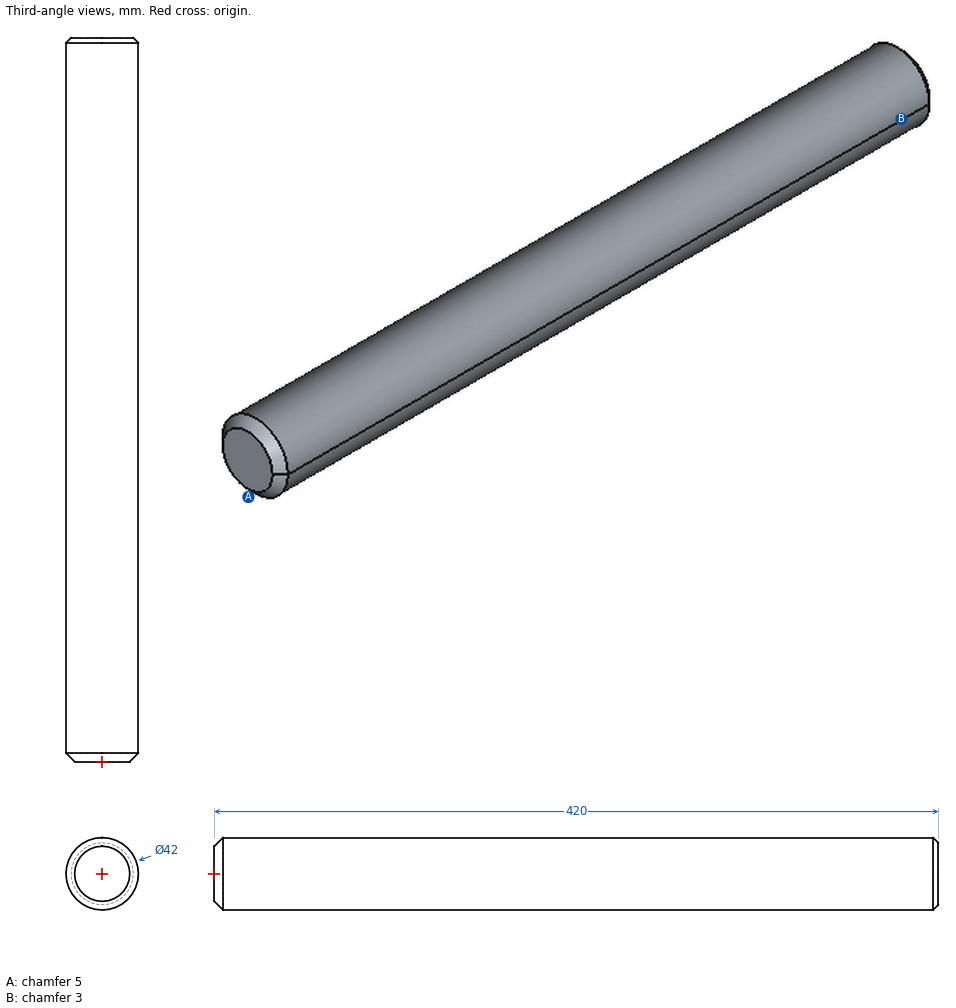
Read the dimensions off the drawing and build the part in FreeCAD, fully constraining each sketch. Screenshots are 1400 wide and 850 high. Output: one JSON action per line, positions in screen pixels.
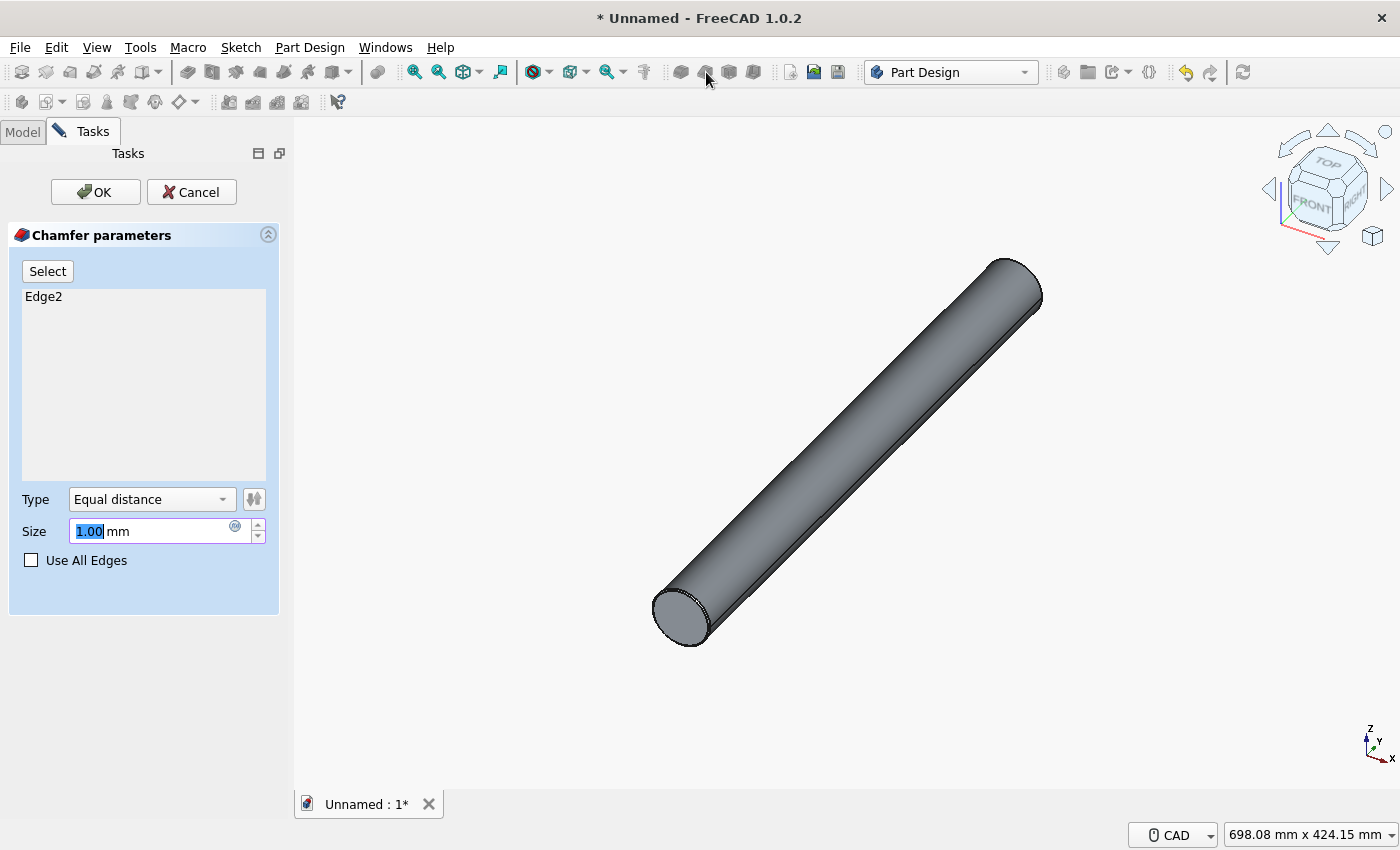
{"action": "type", "text": "5"}
{"action": "key", "text": "Tab"}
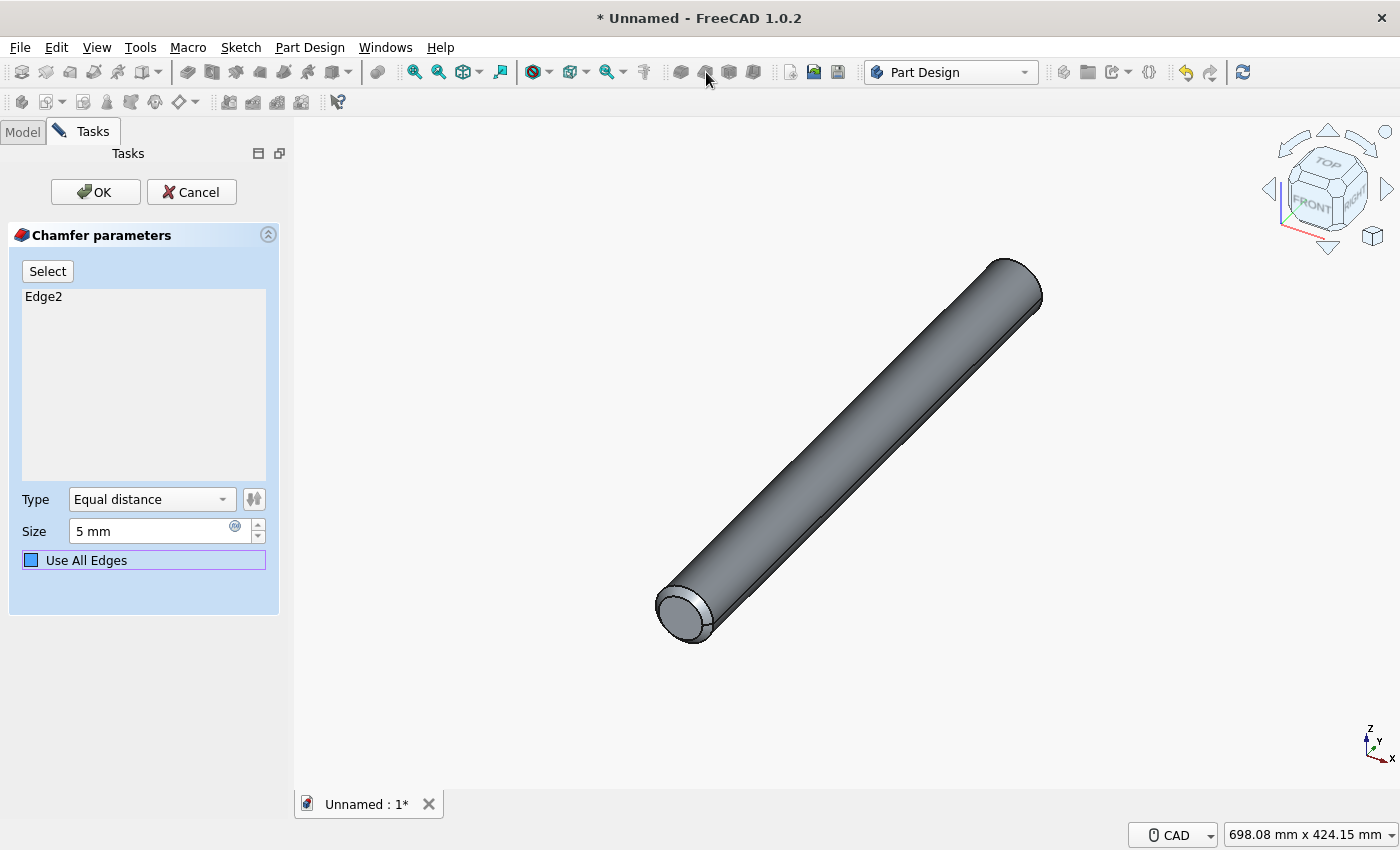
{"action": "left_click", "coordinate": [96, 192]}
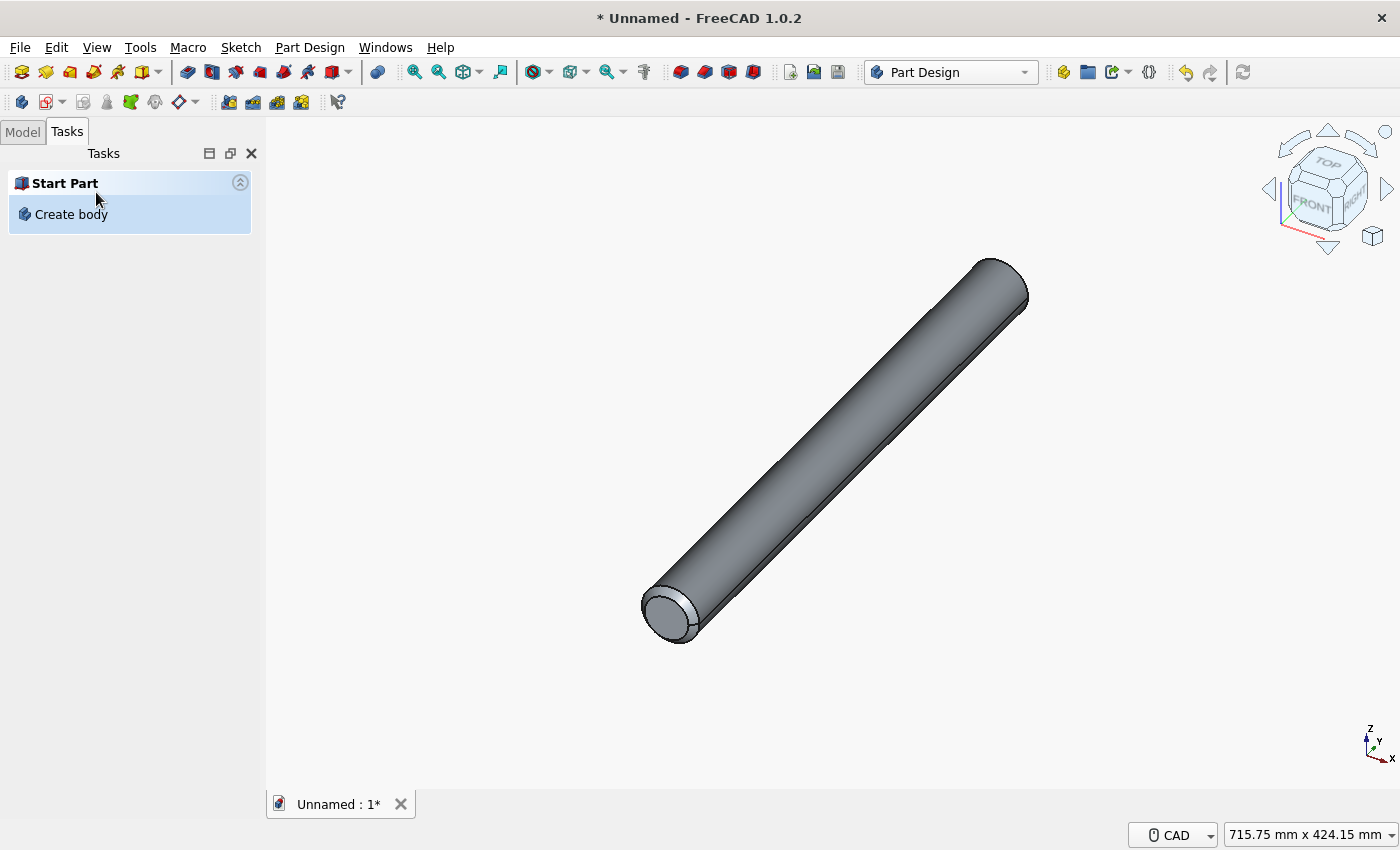
{"action": "key", "text": "0"}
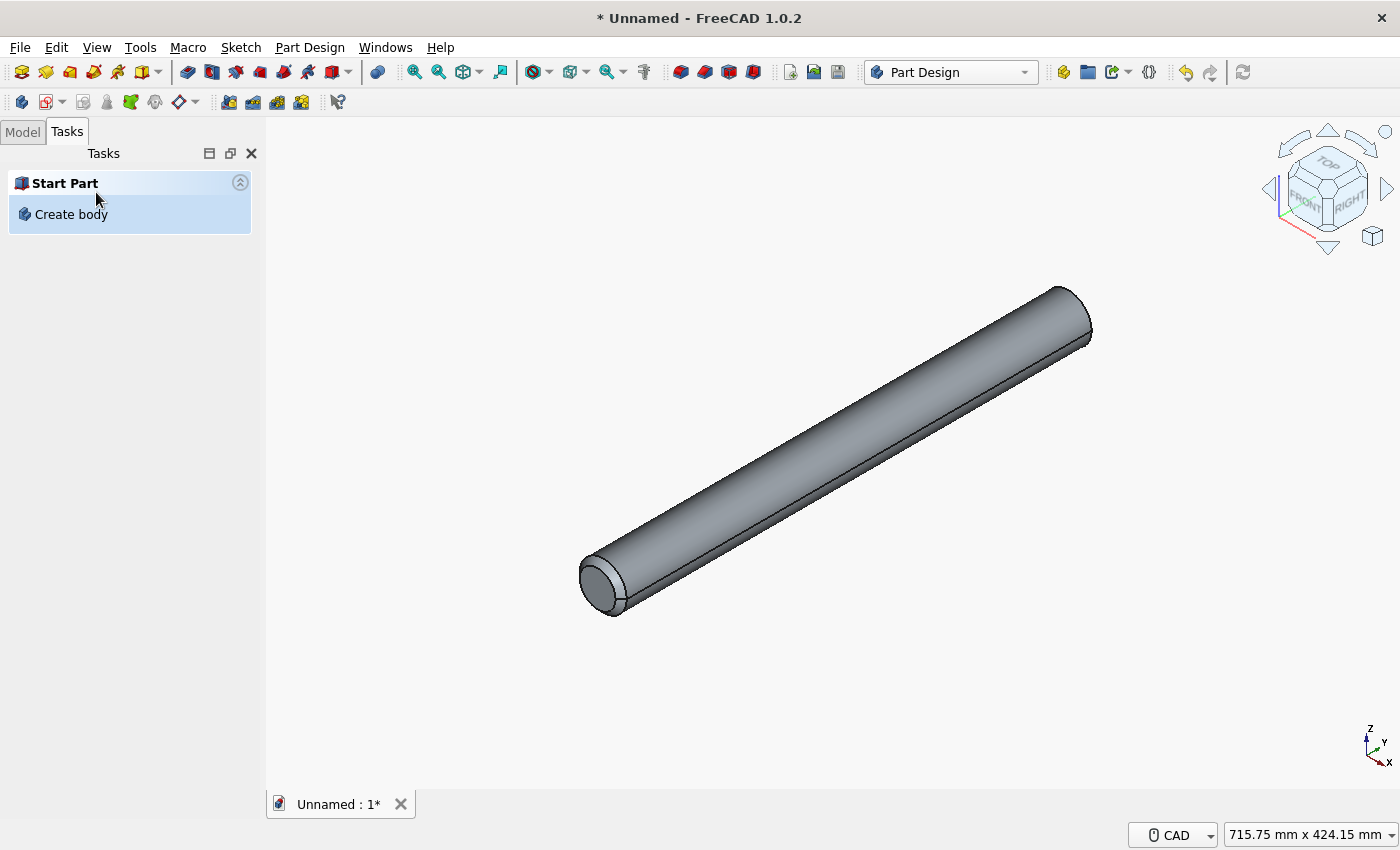
{"action": "key", "text": "2"}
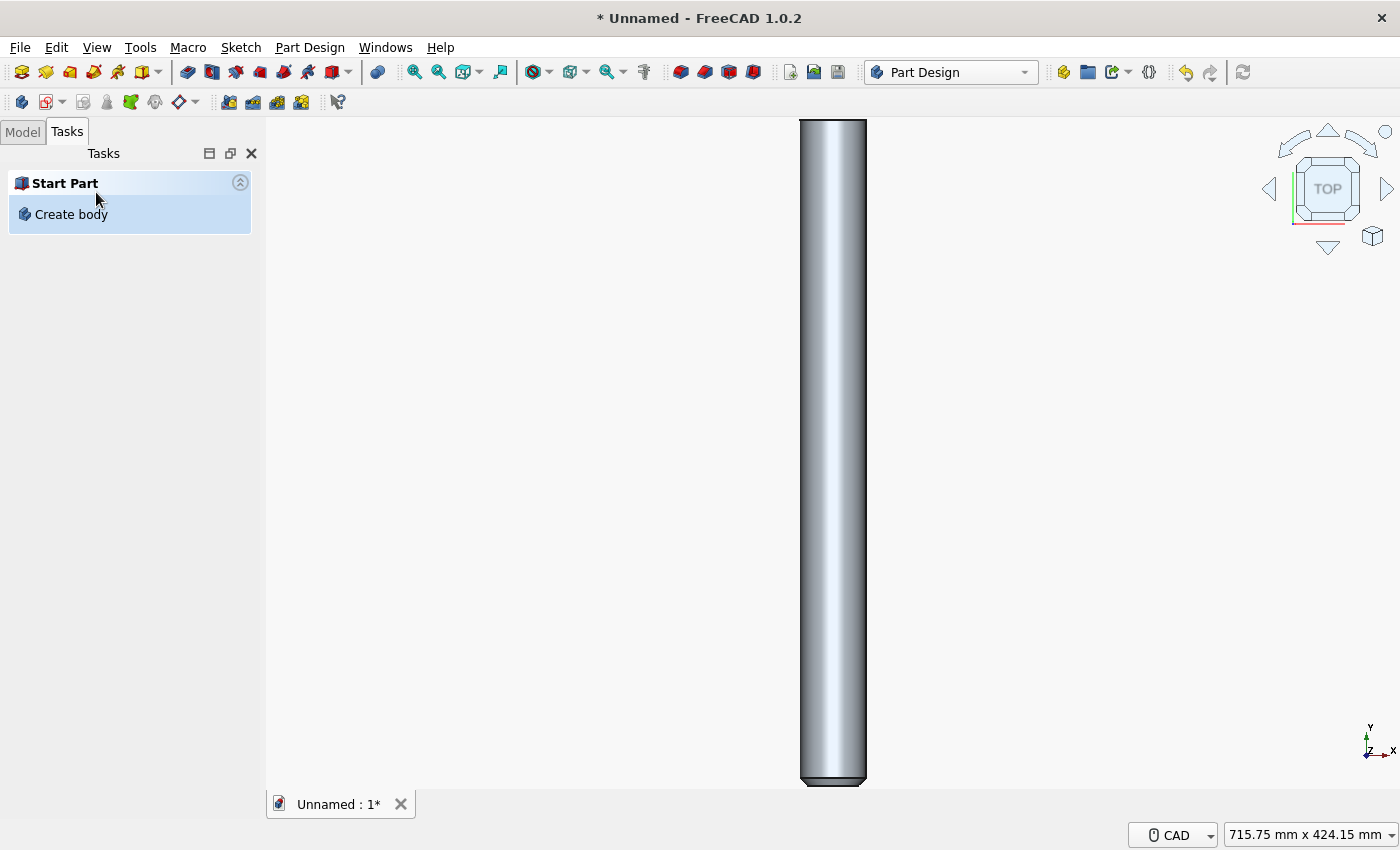
{"action": "key", "text": "1"}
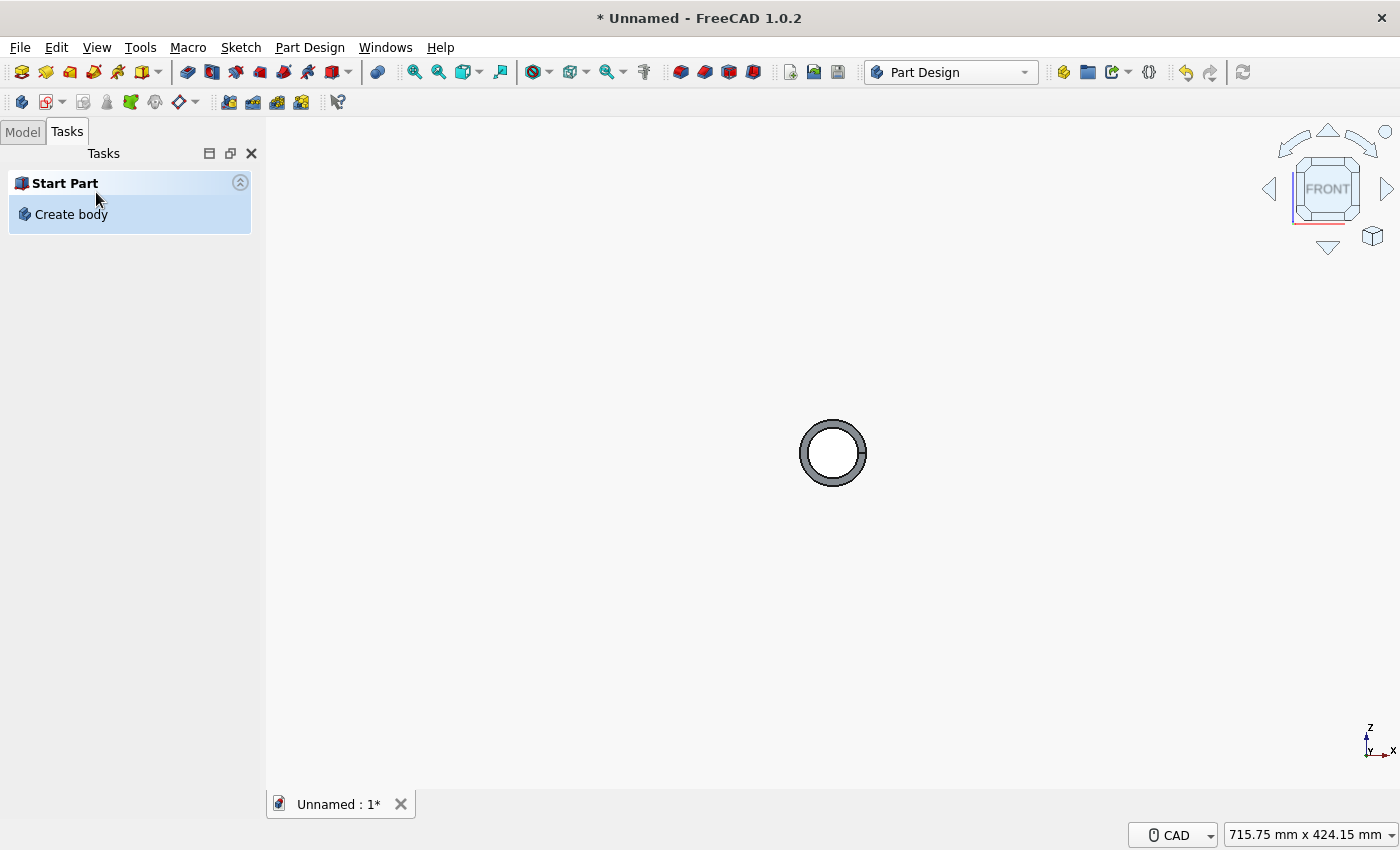
{"action": "key", "text": "v f"}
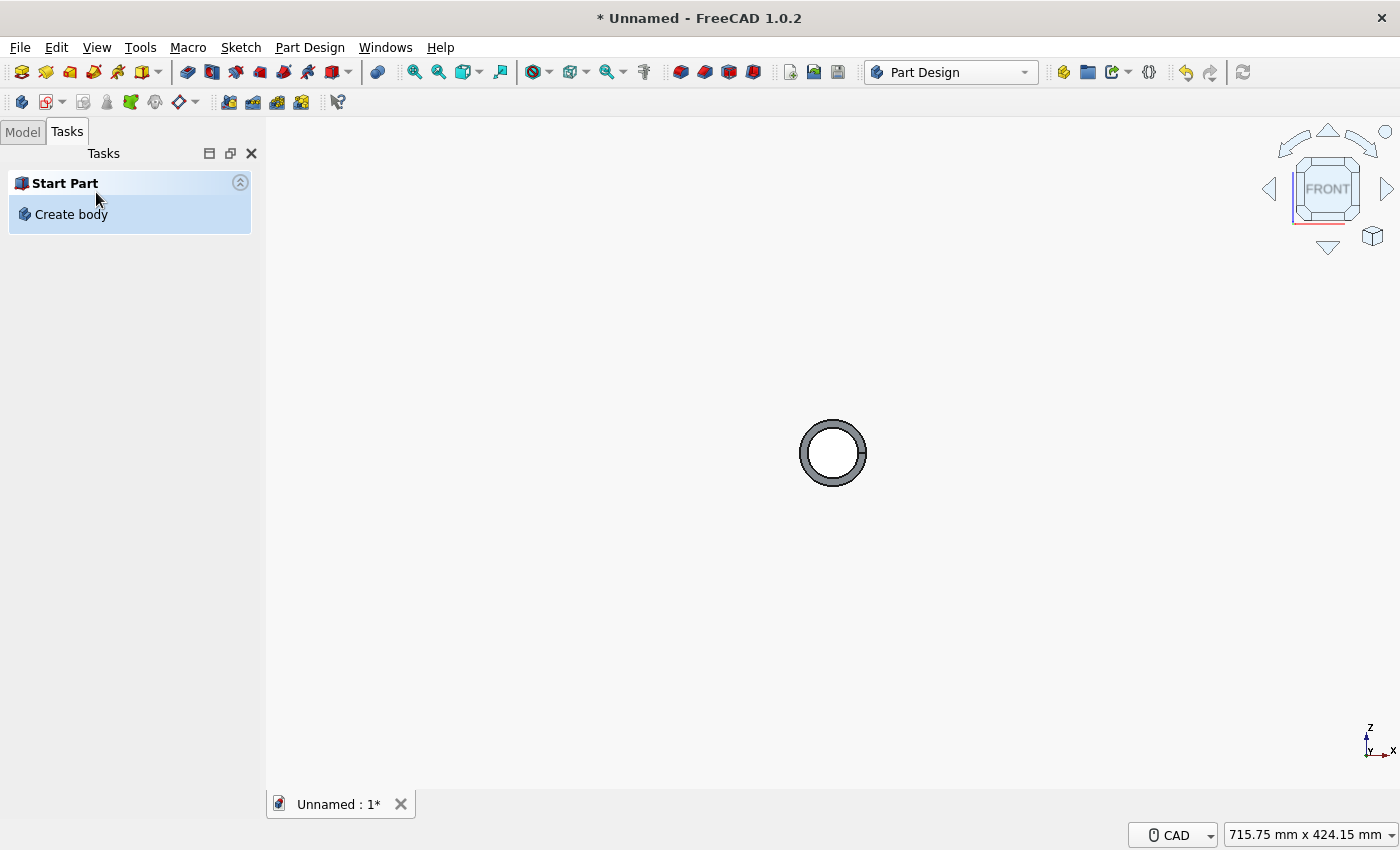
{"action": "key", "text": "3"}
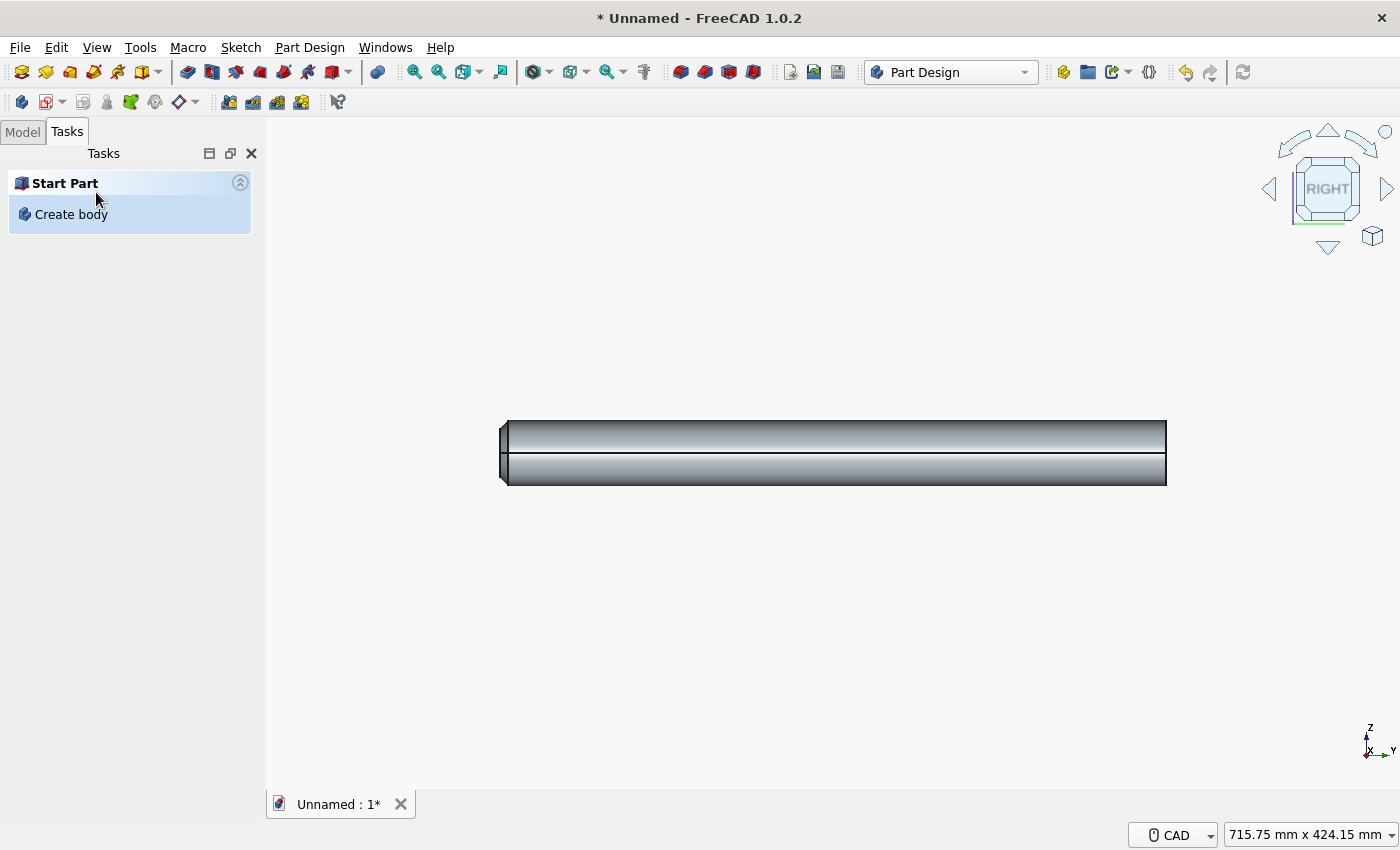
{"action": "left_click", "coordinate": [1166, 432]}